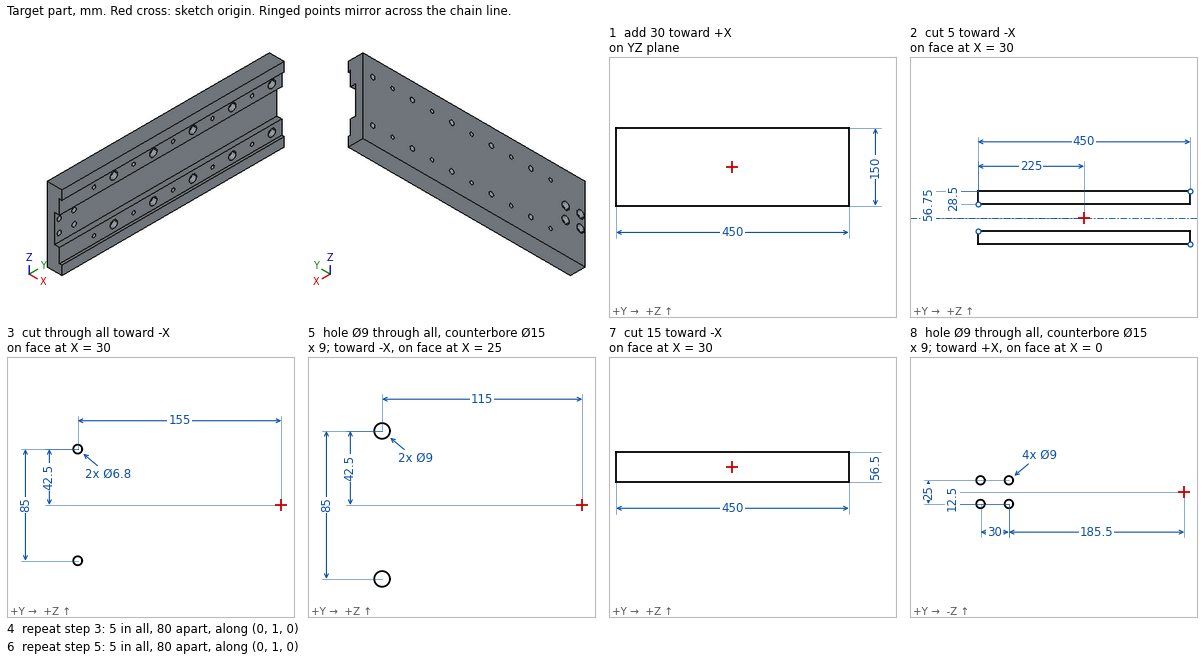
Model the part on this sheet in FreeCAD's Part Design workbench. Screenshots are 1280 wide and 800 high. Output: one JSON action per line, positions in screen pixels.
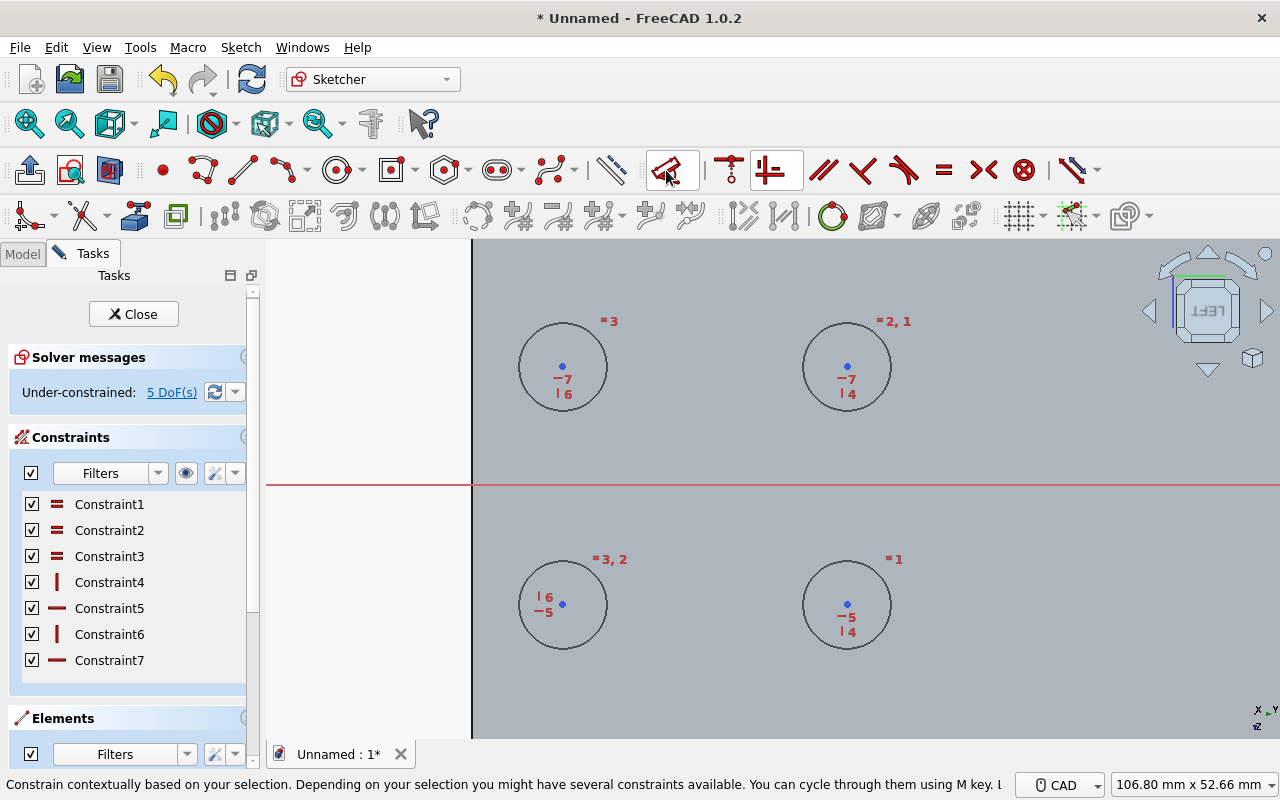
{"action": "left_click", "coordinate": [878, 574]}
{"action": "left_click", "coordinate": [901, 551]}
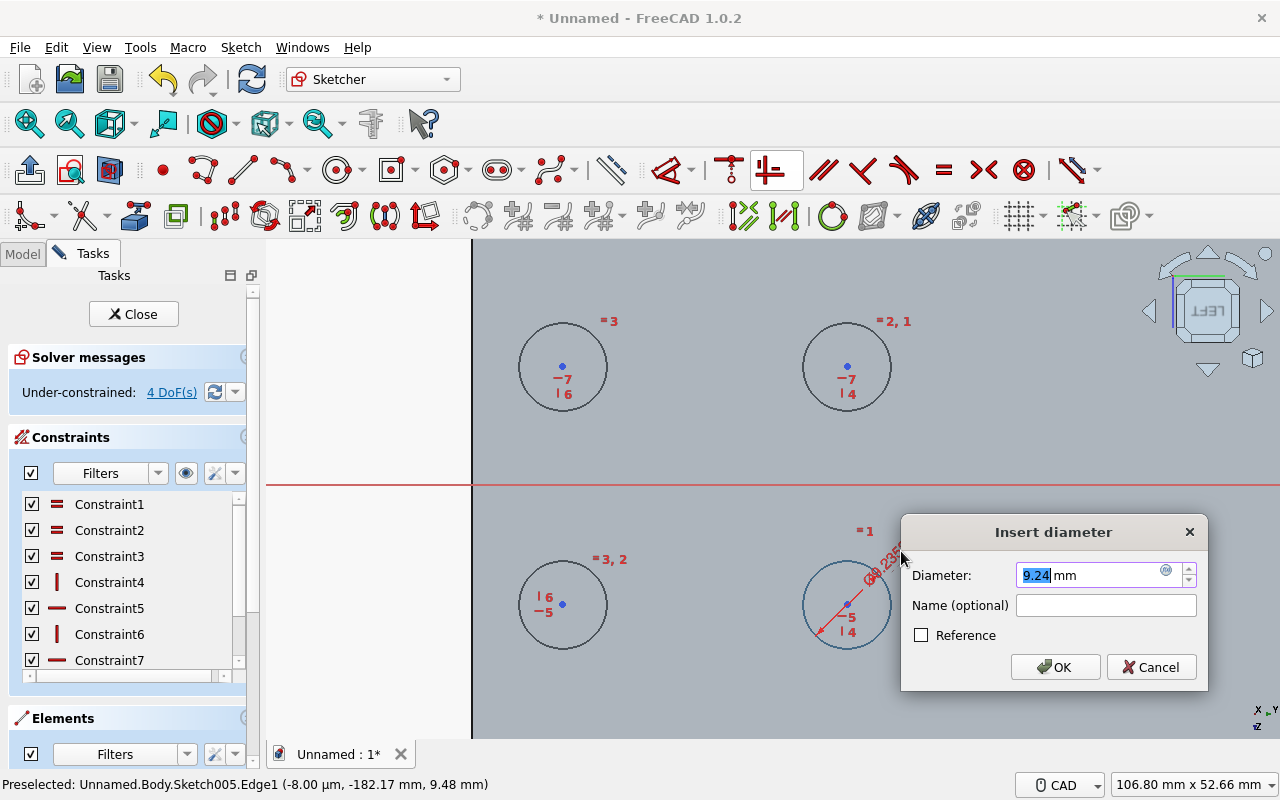
{"action": "type", "text": "9"}
{"action": "key", "text": "Return"}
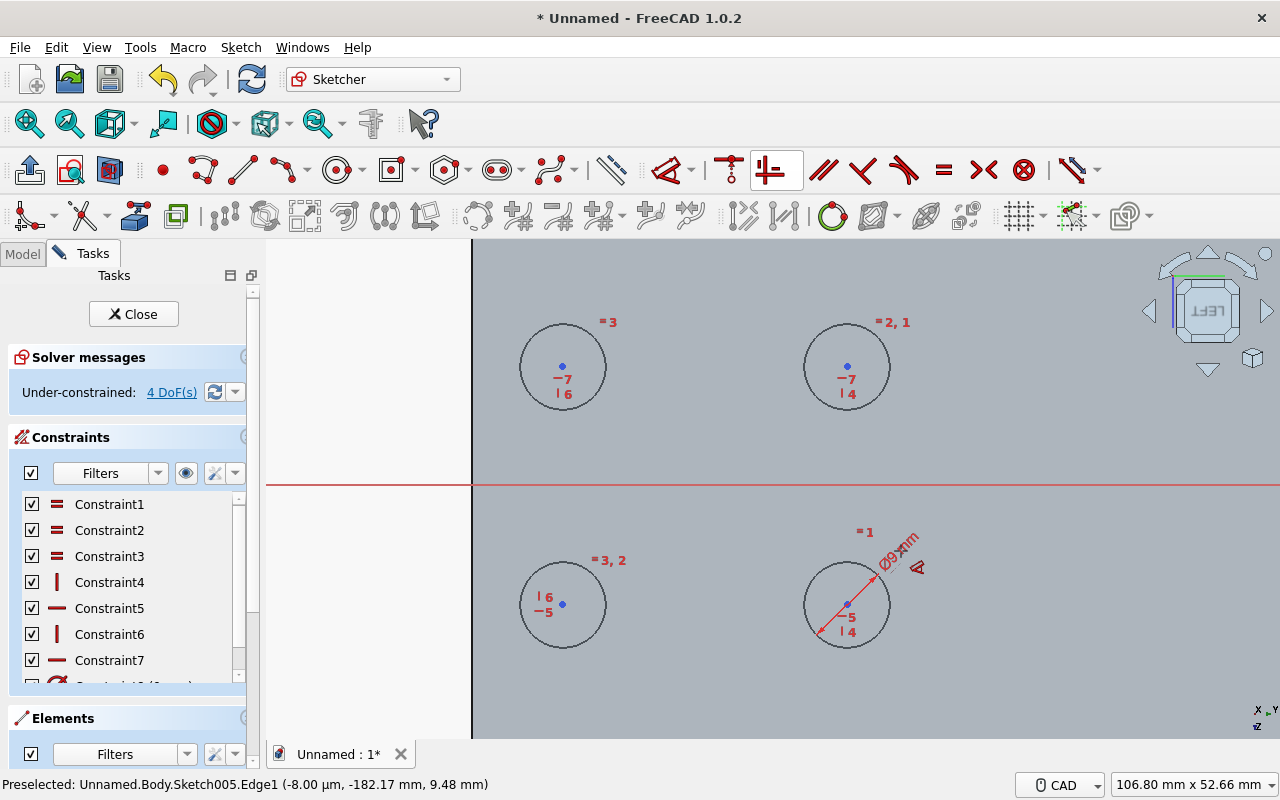
{"action": "left_click", "coordinate": [847, 605]}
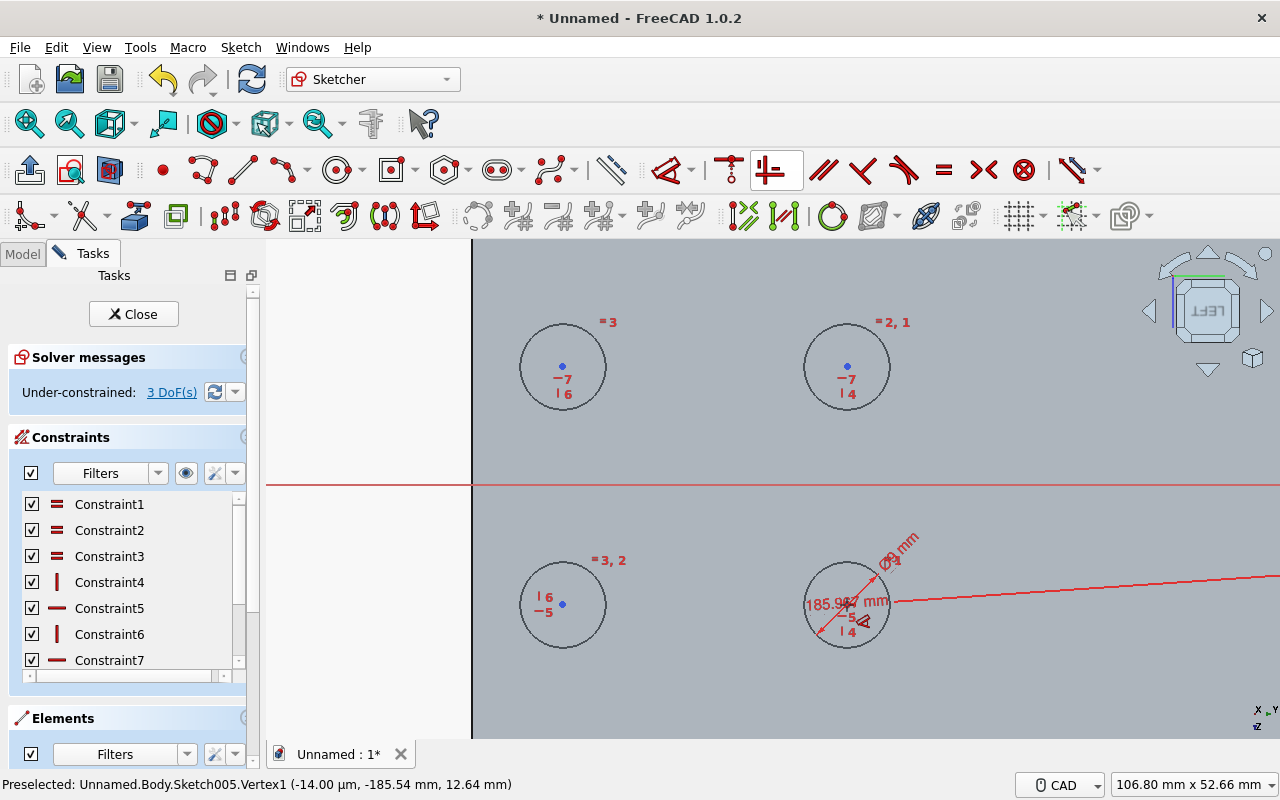
{"action": "left_click", "coordinate": [847, 367]}
{"action": "left_click", "coordinate": [881, 431]}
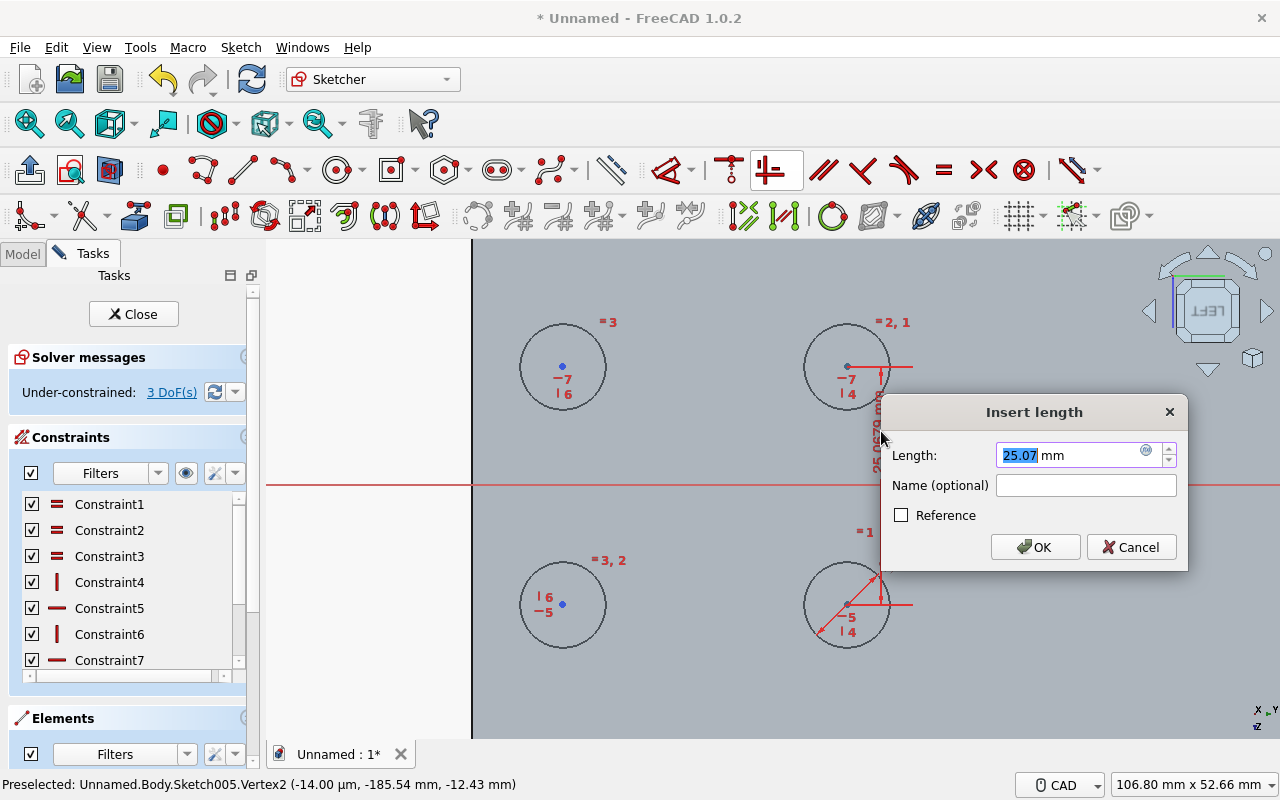
{"action": "type", "text": "25"}
{"action": "key", "text": "Return"}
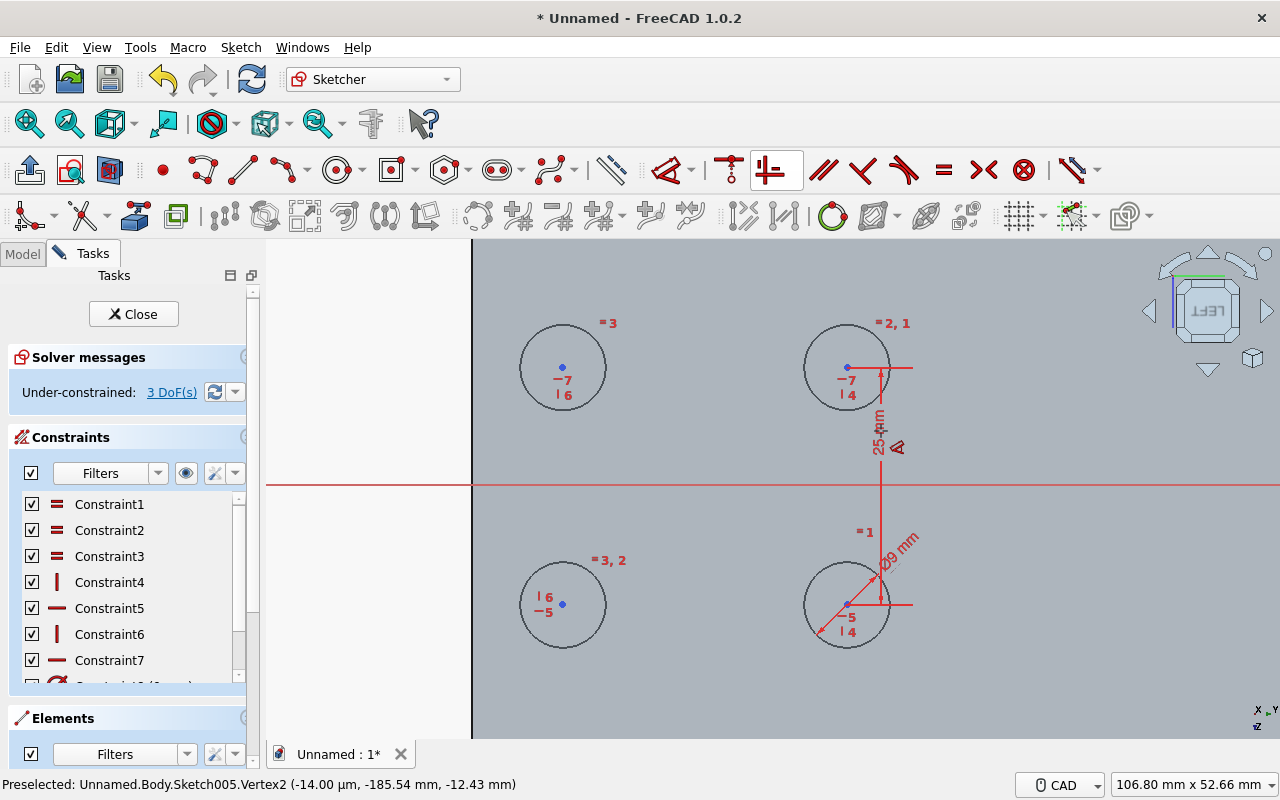
{"action": "left_click", "coordinate": [847, 605]}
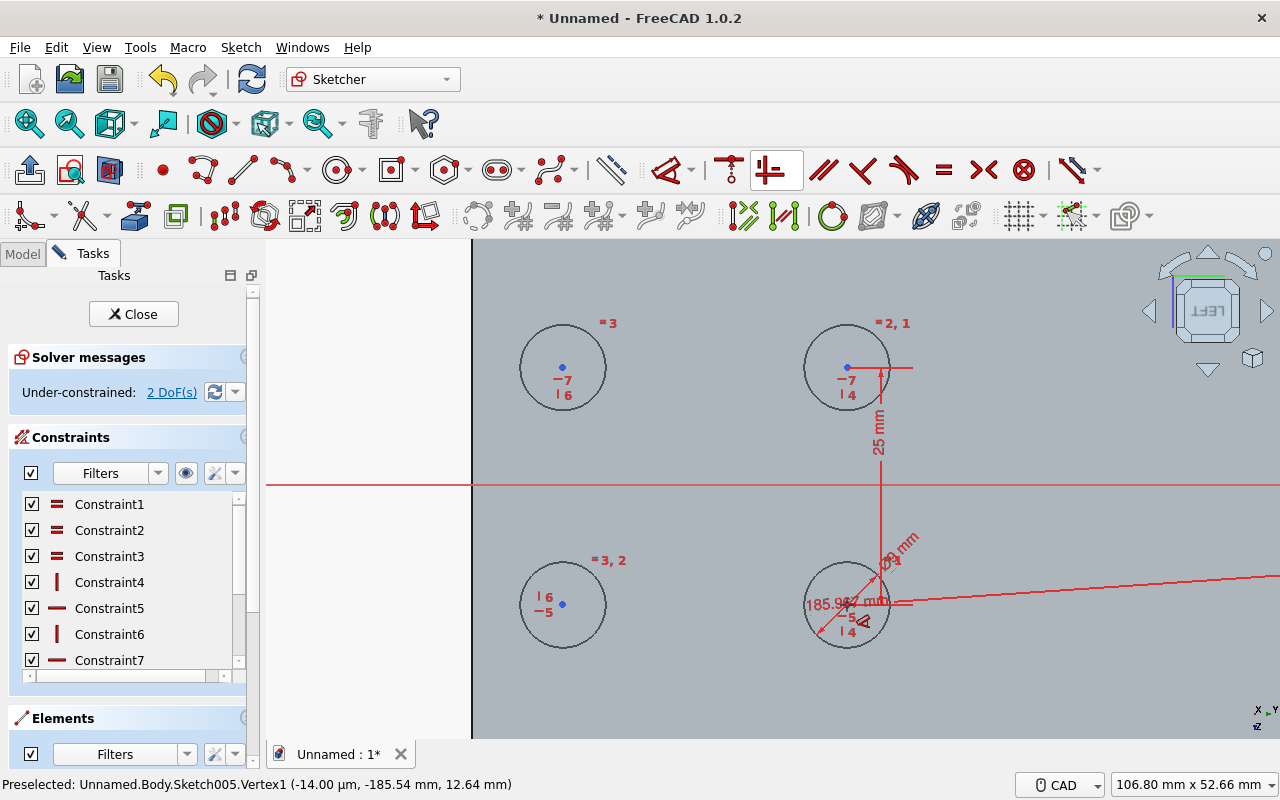
{"action": "left_click", "coordinate": [563, 605]}
{"action": "left_click", "coordinate": [705, 639]}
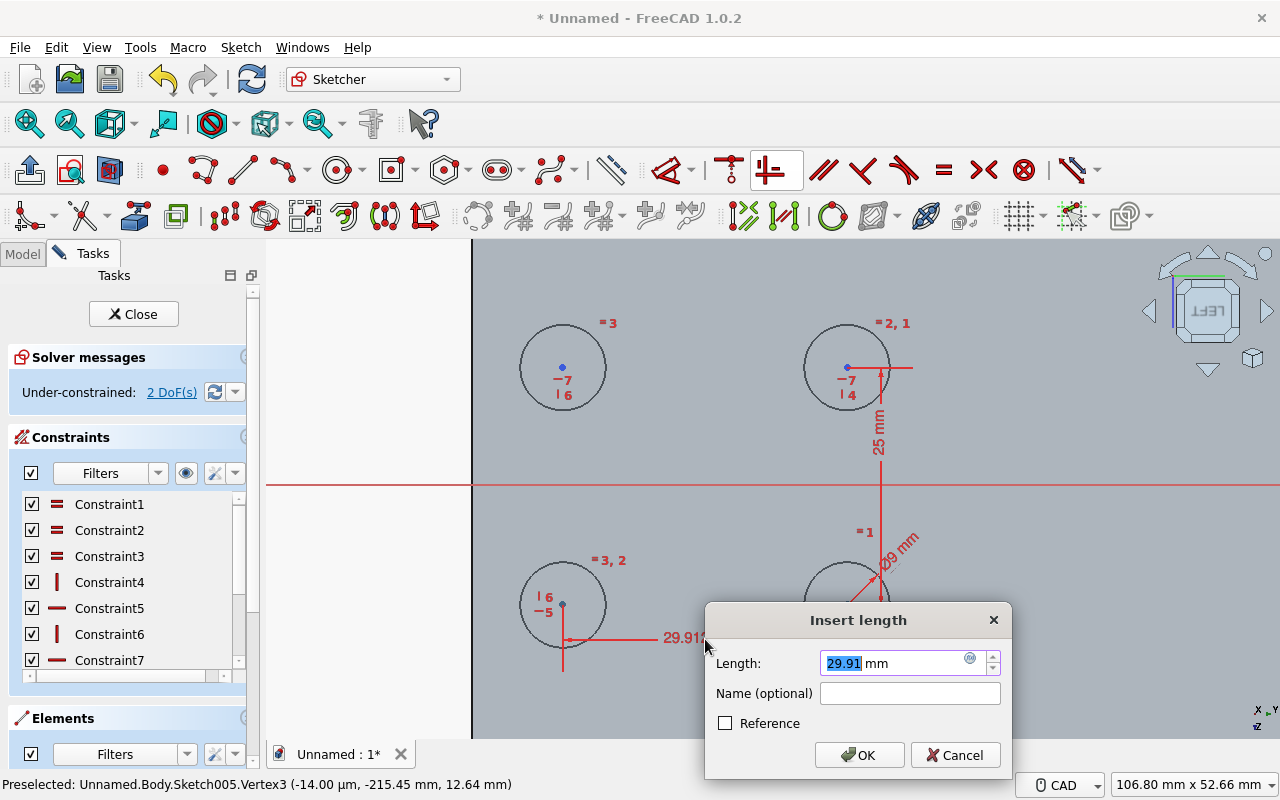
{"action": "type", "text": "30"}
{"action": "key", "text": "Return"}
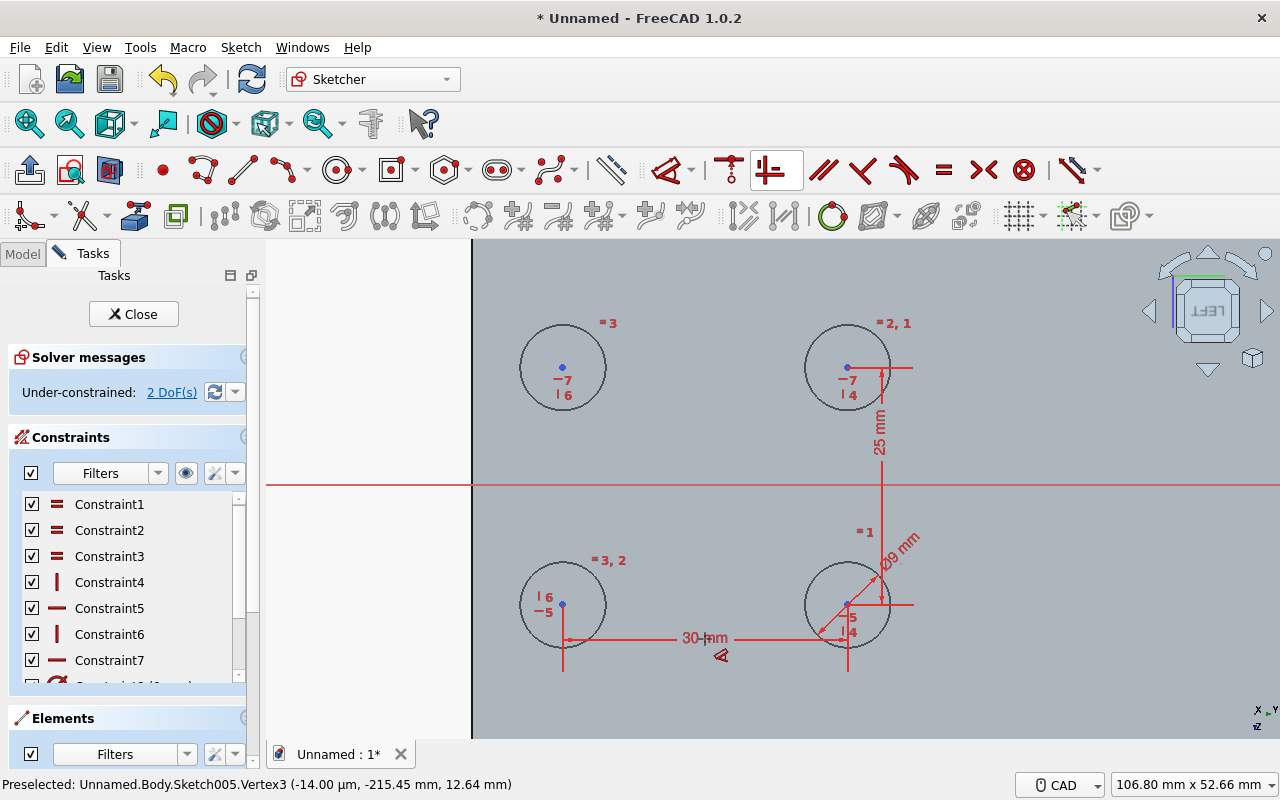
{"action": "left_click", "coordinate": [848, 605]}
{"action": "left_click", "coordinate": [814, 545]}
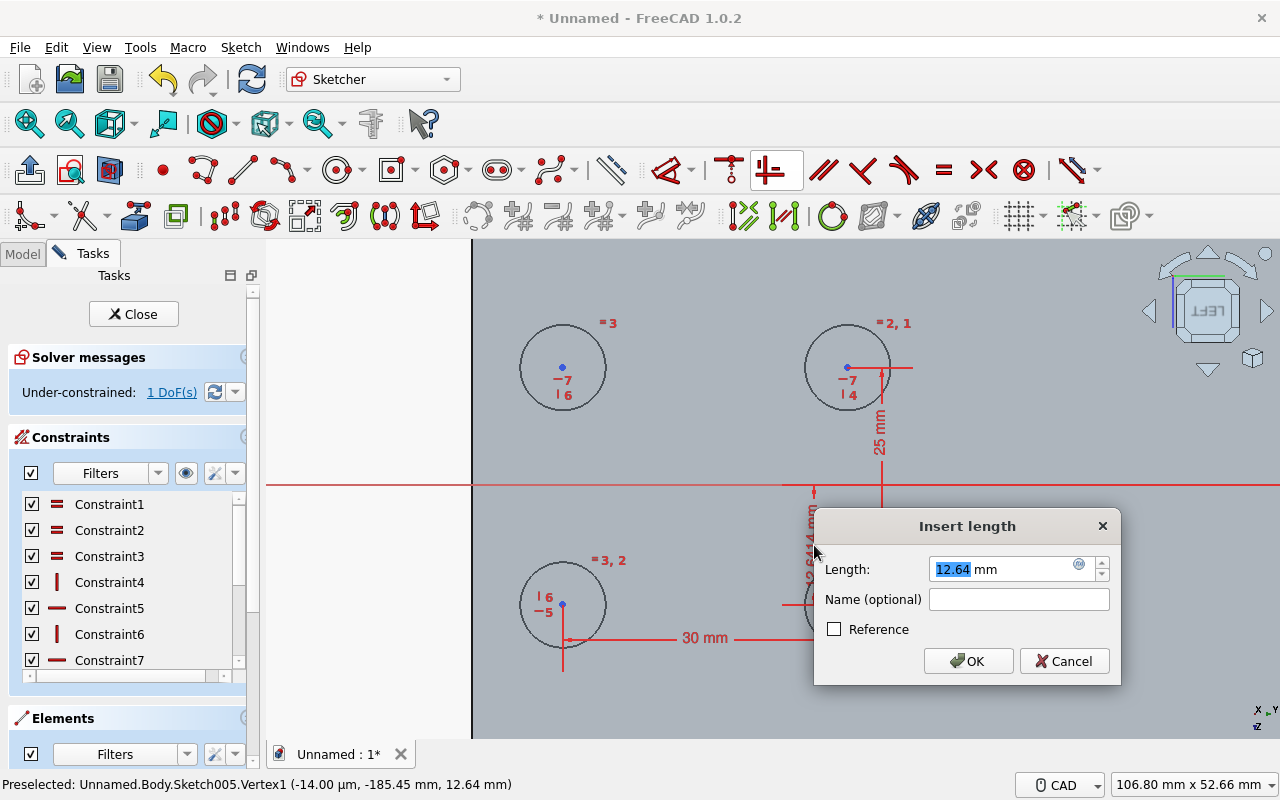
{"action": "type", "text": "12.5"}
{"action": "key", "text": "Return"}